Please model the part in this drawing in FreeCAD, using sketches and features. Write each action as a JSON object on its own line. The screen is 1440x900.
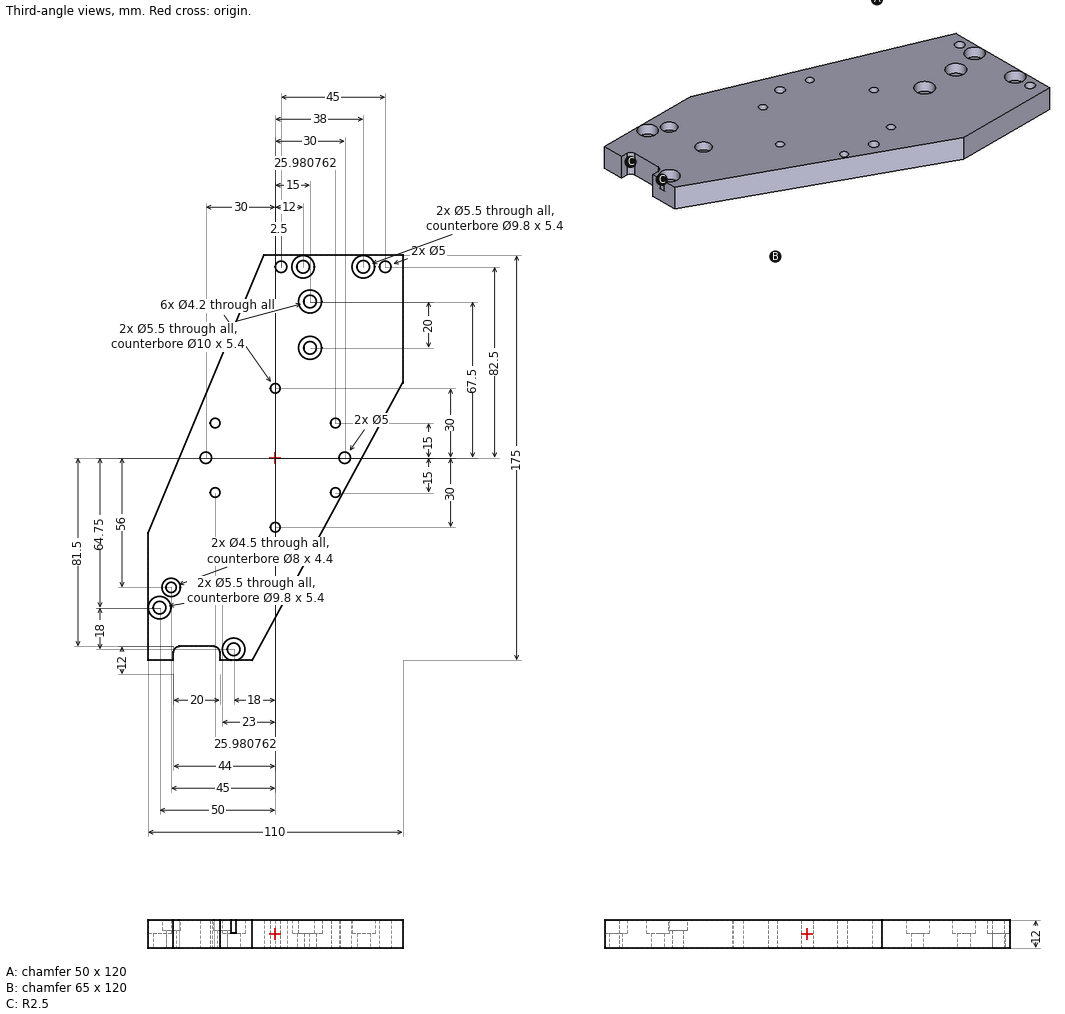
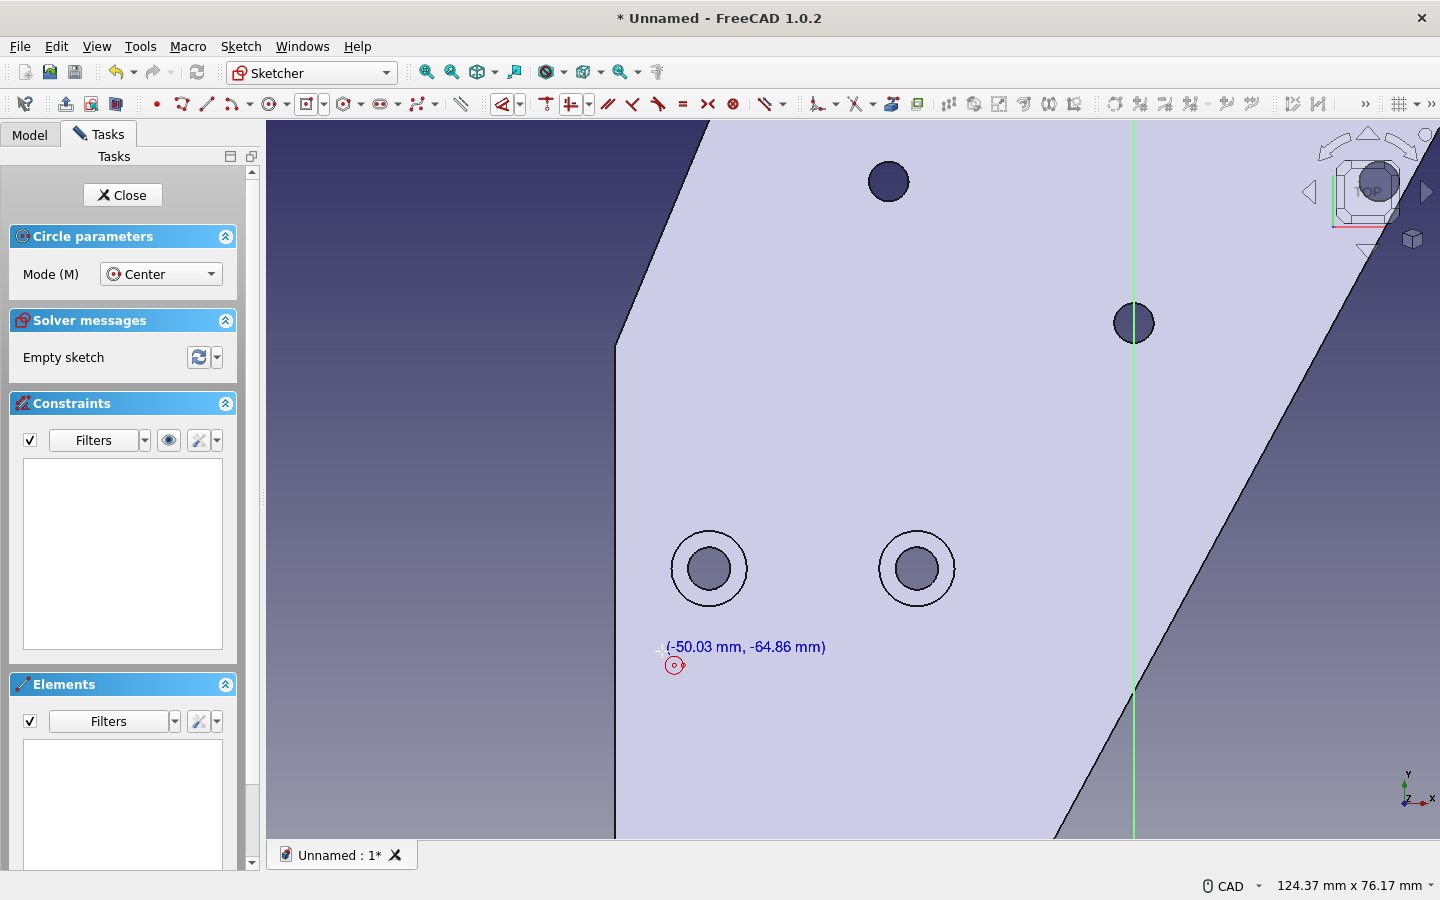
{"action": "left_click", "coordinate": [662, 651]}
{"action": "left_click", "coordinate": [680, 633]}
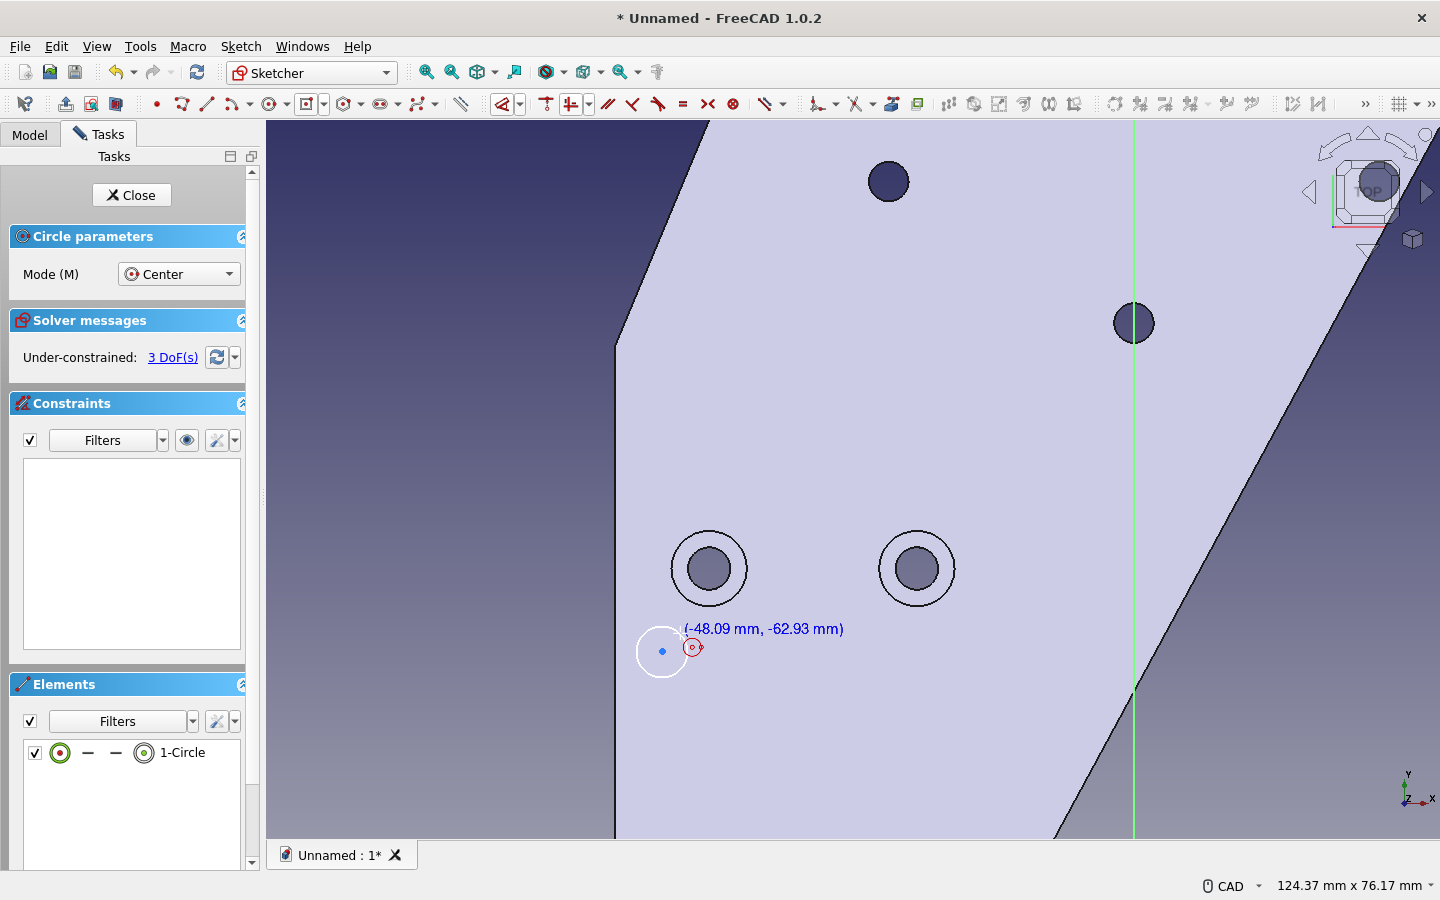
{"action": "scroll", "coordinate": [662, 523], "scroll_direction": "down", "scroll_amount": 3}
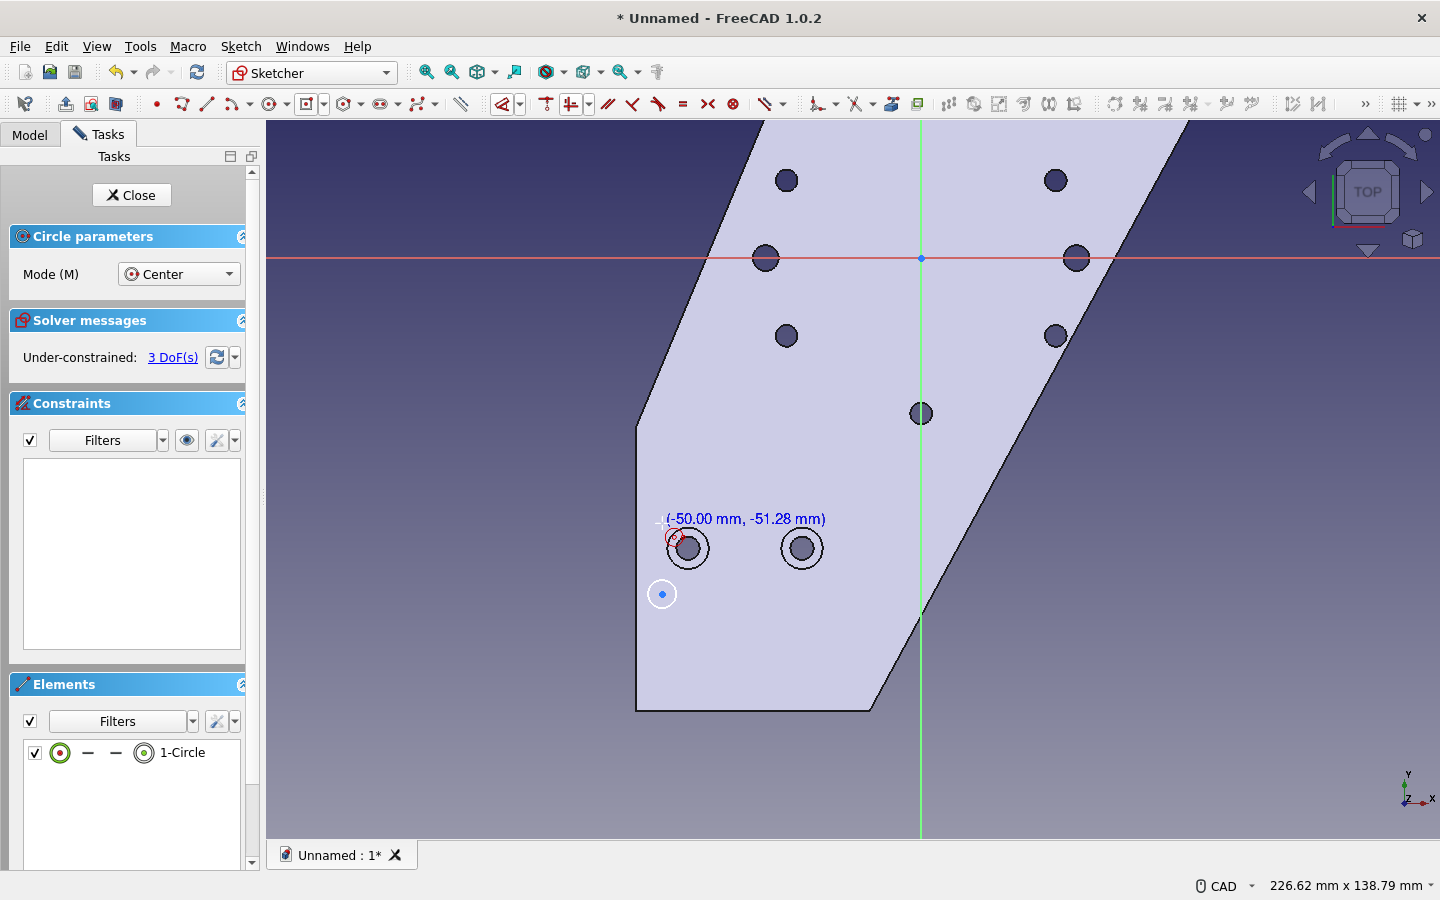
{"action": "scroll", "coordinate": [828, 687], "scroll_direction": "up", "scroll_amount": 3}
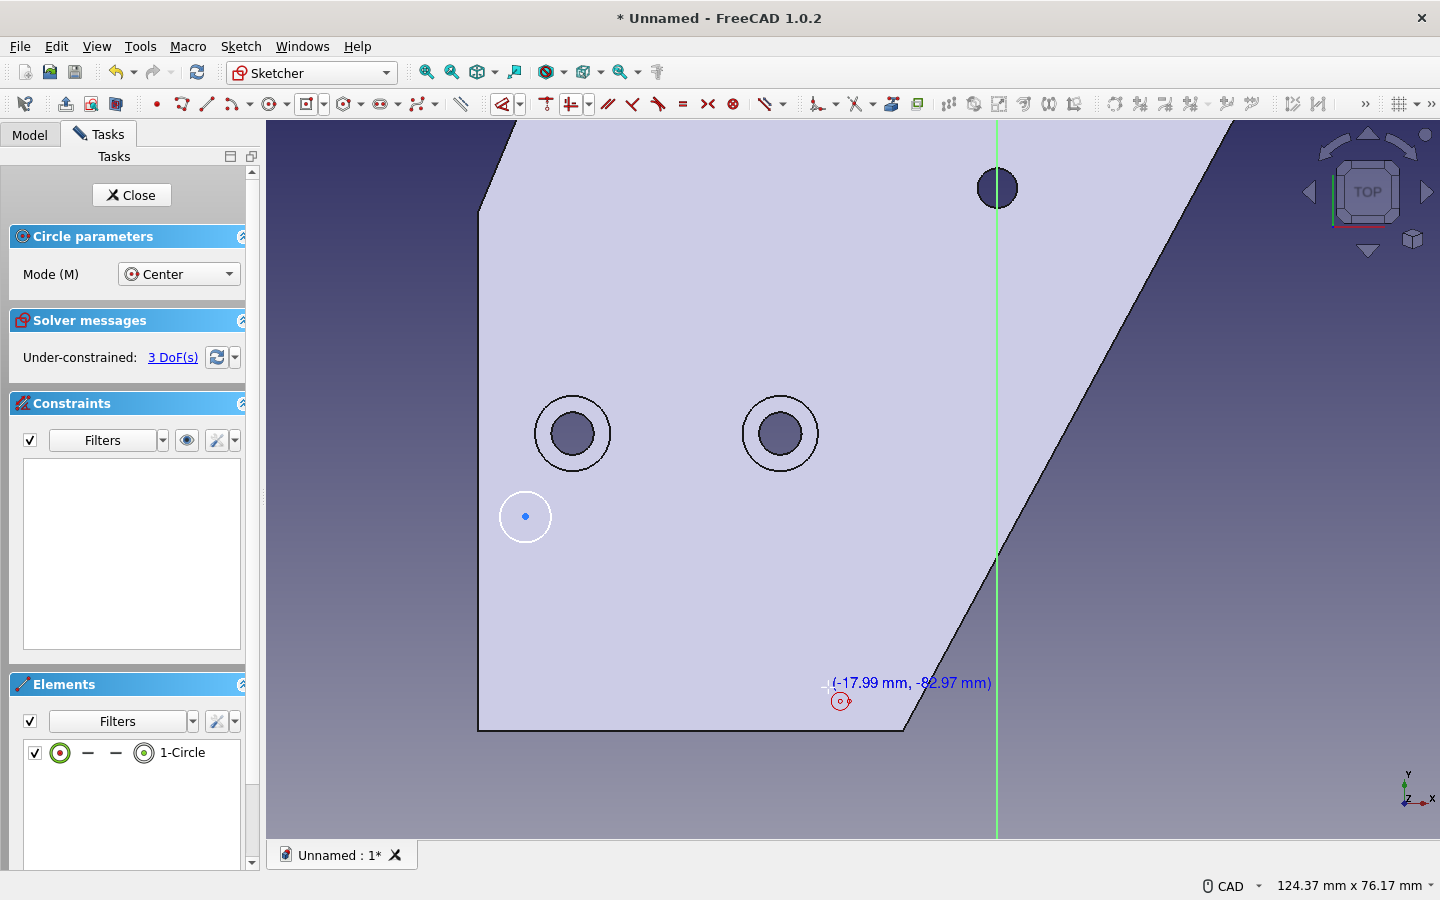
{"action": "left_click", "coordinate": [827, 686]}
{"action": "left_click", "coordinate": [846, 668]}
{"action": "key", "text": "Escape"}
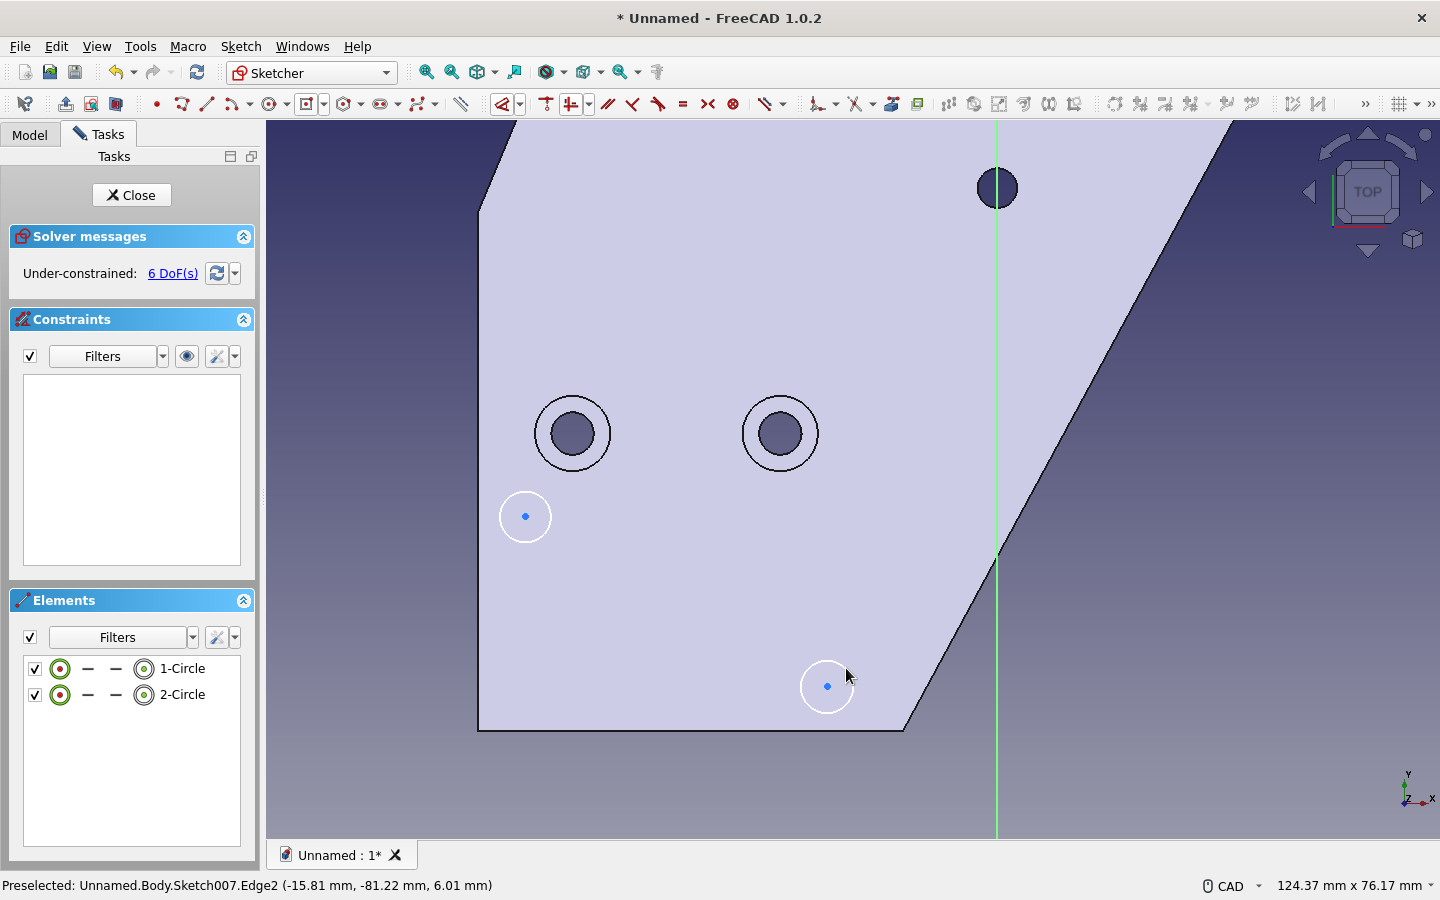
{"action": "left_click", "coordinate": [543, 499]}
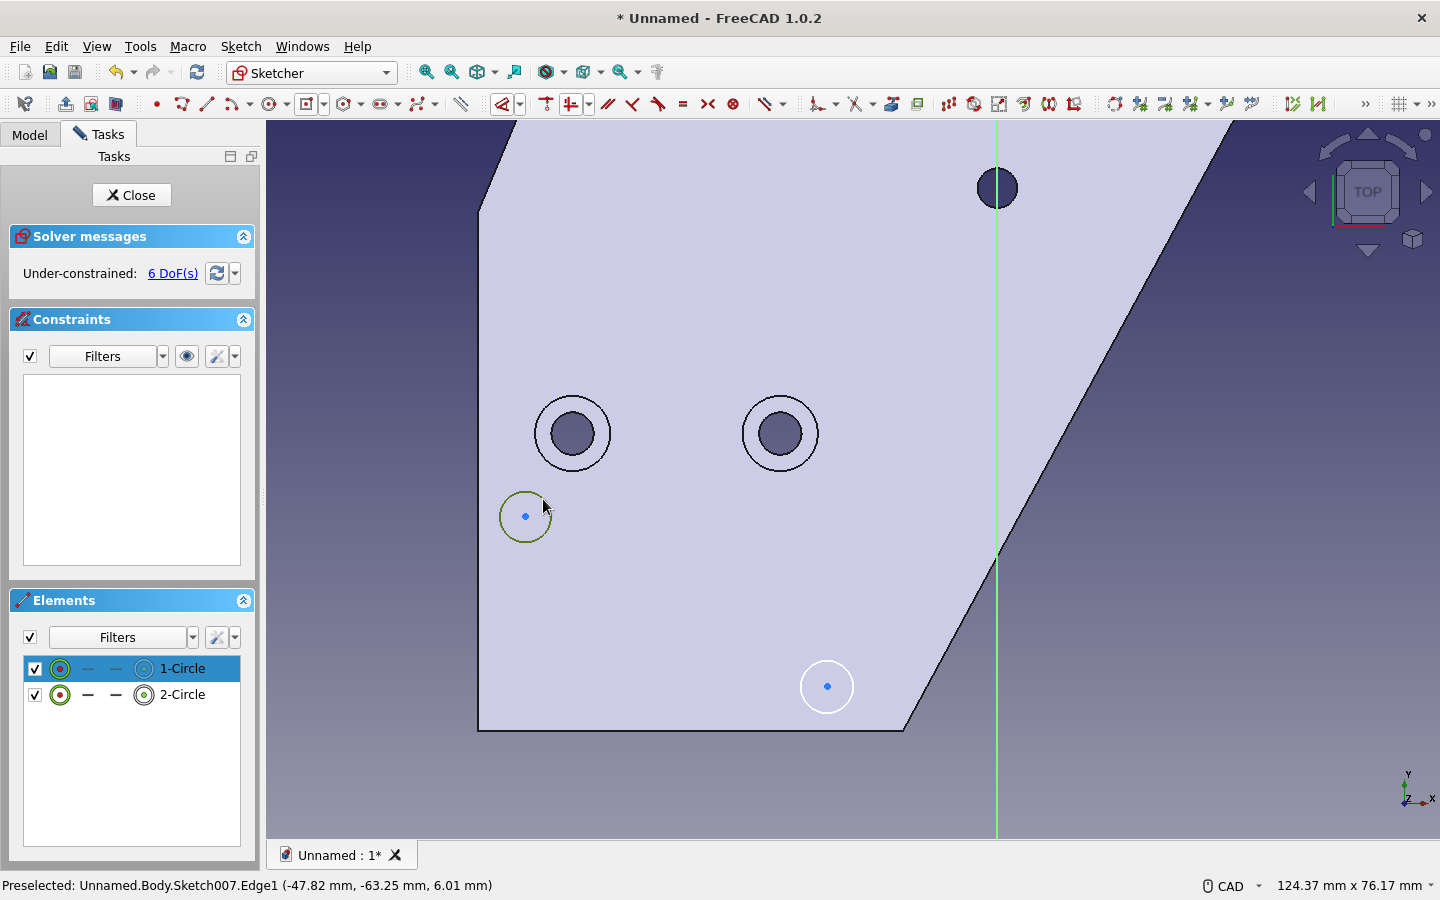
{"action": "left_click", "coordinate": [845, 668]}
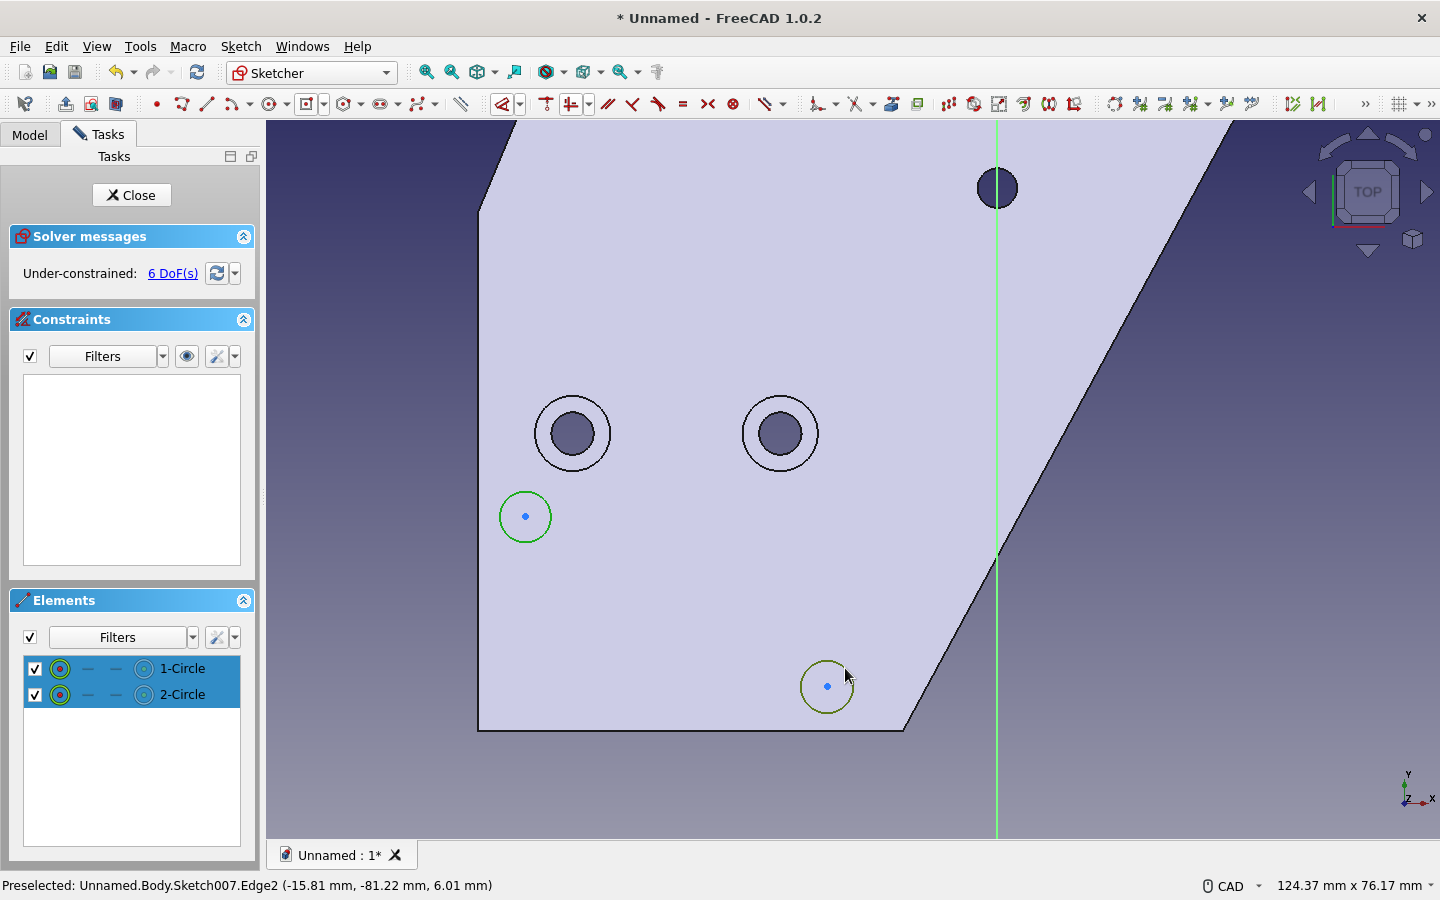
{"action": "left_click", "coordinate": [683, 104]}